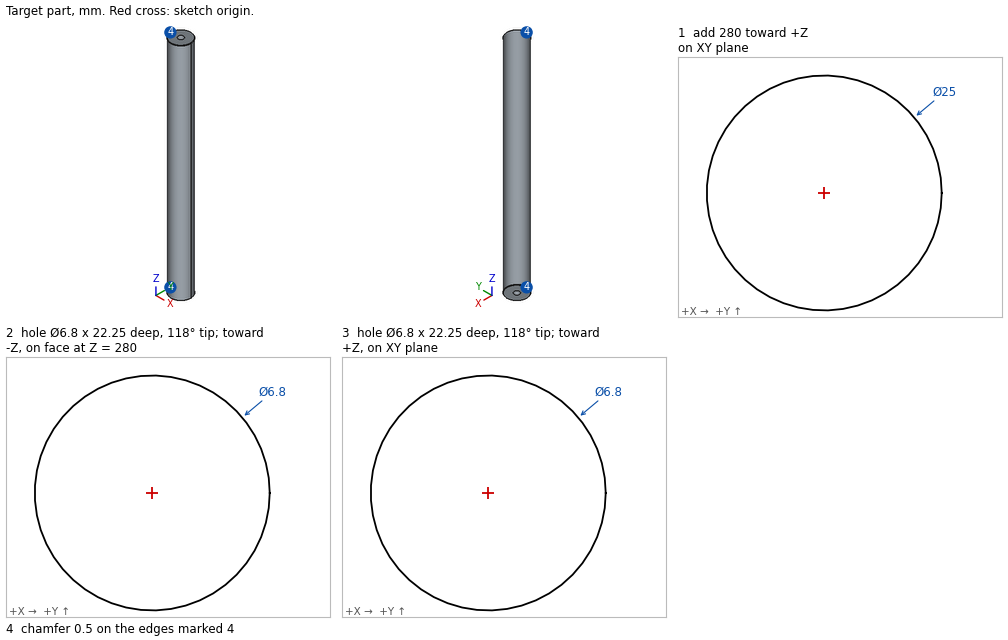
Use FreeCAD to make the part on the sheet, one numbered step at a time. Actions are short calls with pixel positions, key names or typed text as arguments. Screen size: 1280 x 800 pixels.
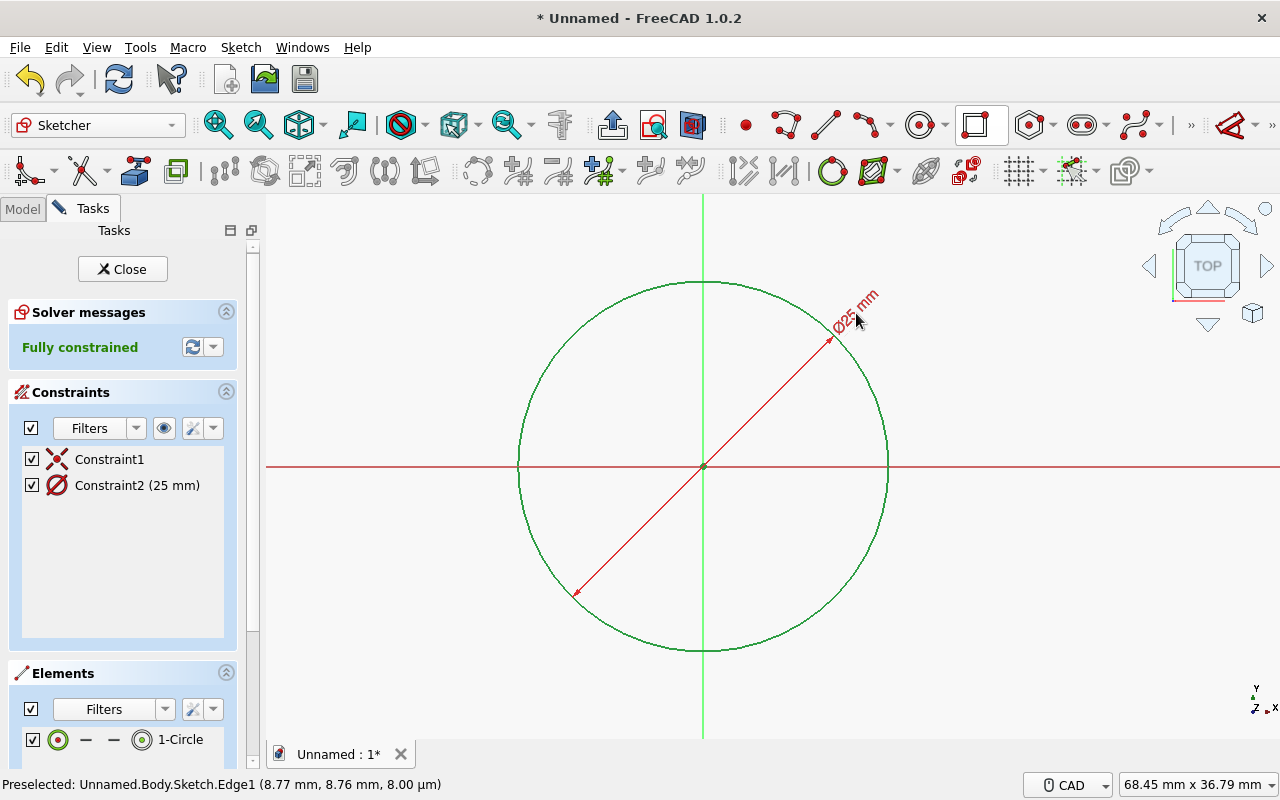
click(123, 269)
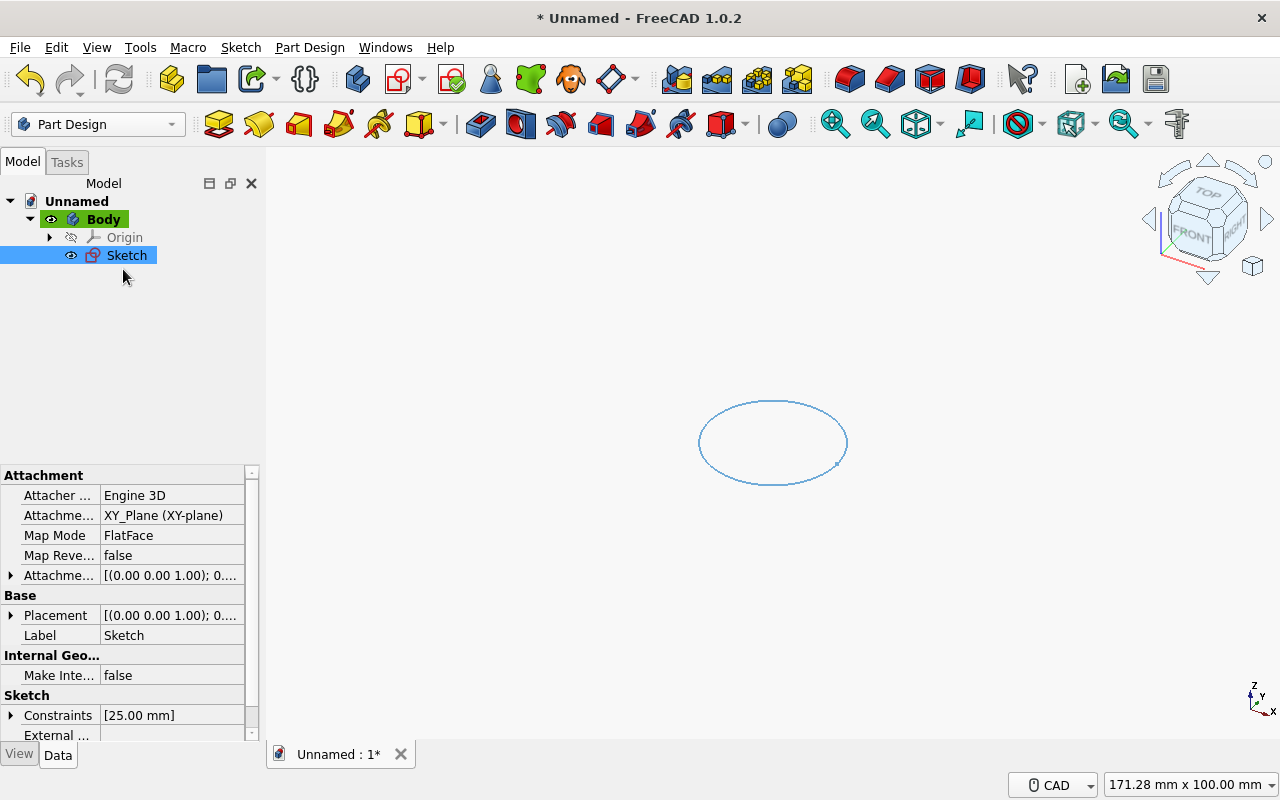
click(220, 124)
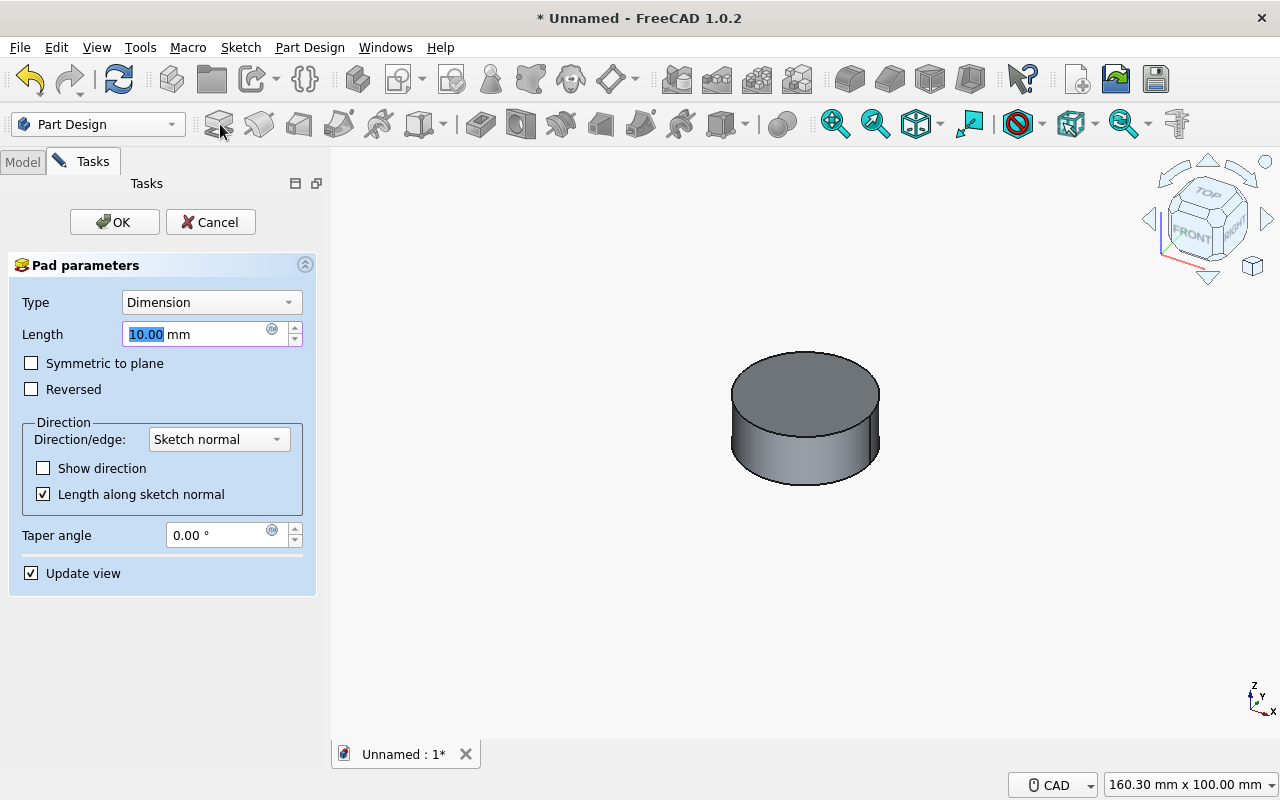
text(280)
key(Tab)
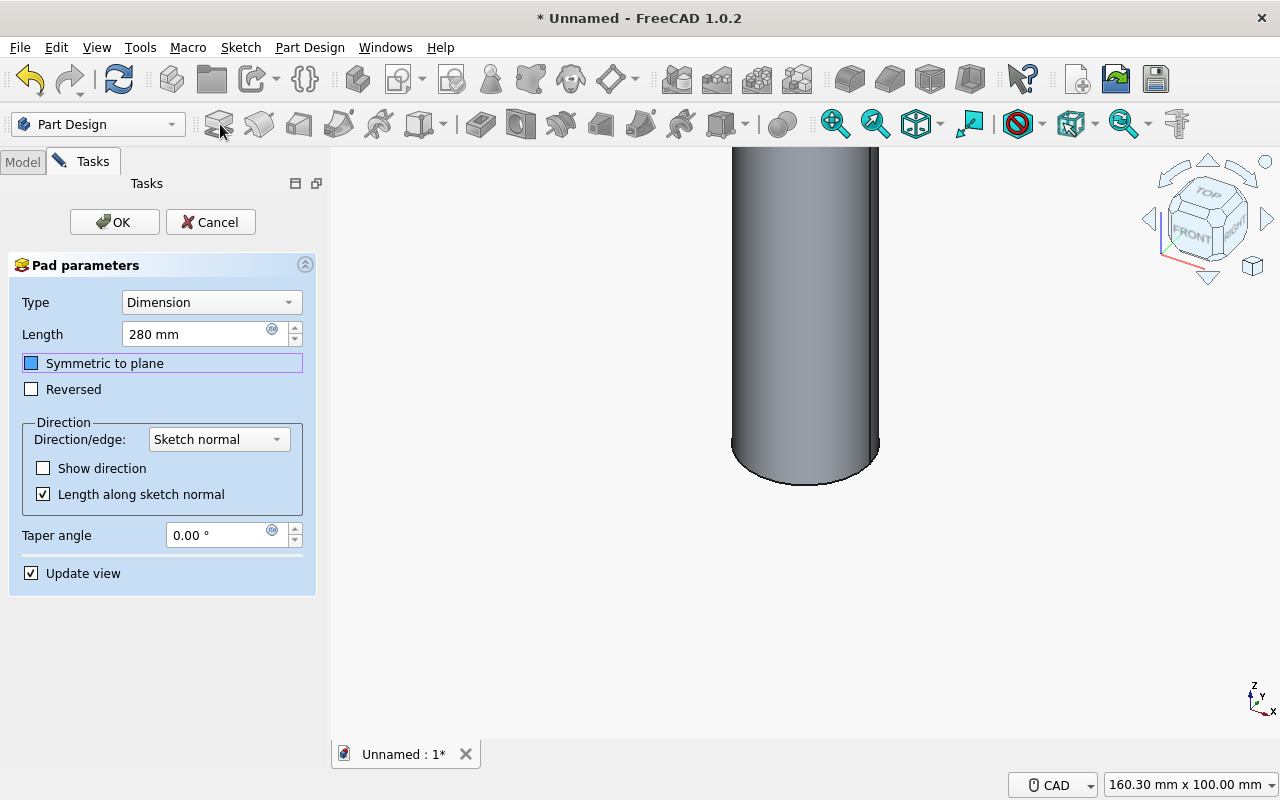
click(115, 222)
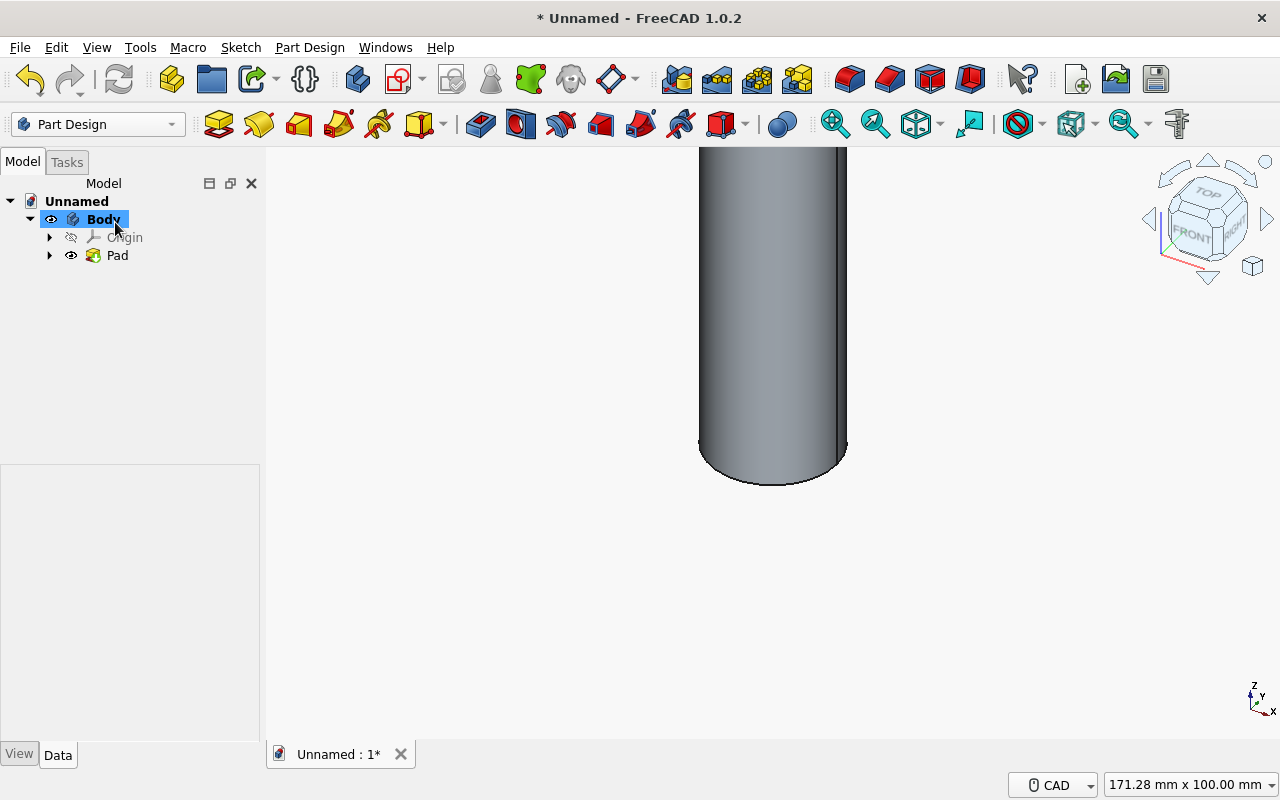
click(836, 124)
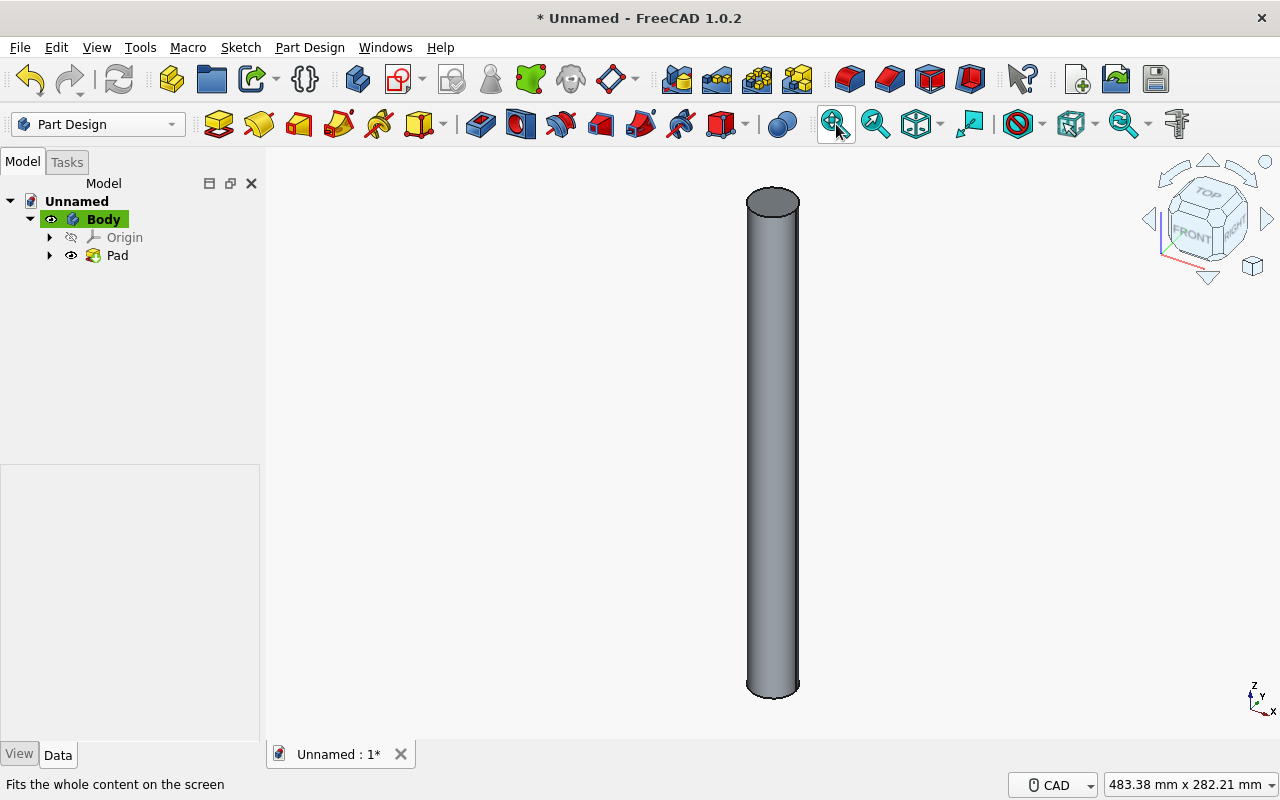
click(773, 201)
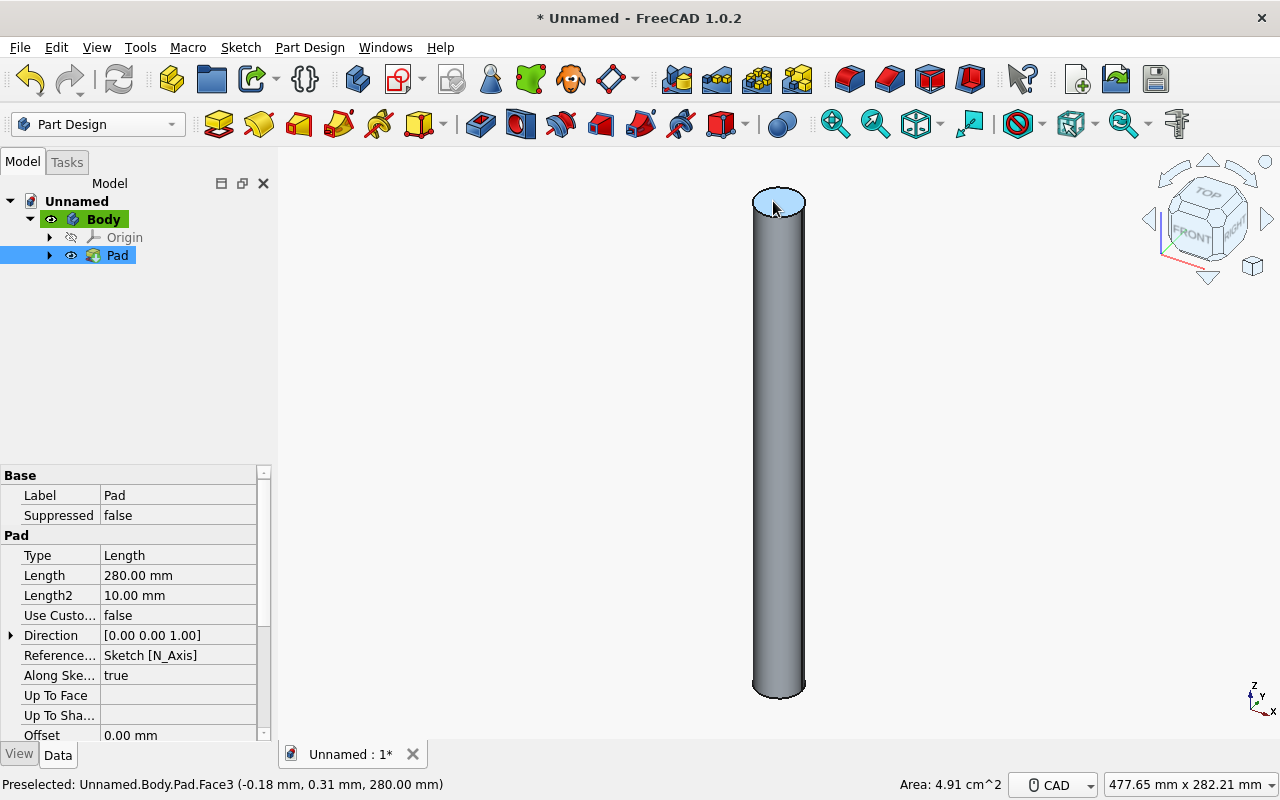
click(398, 80)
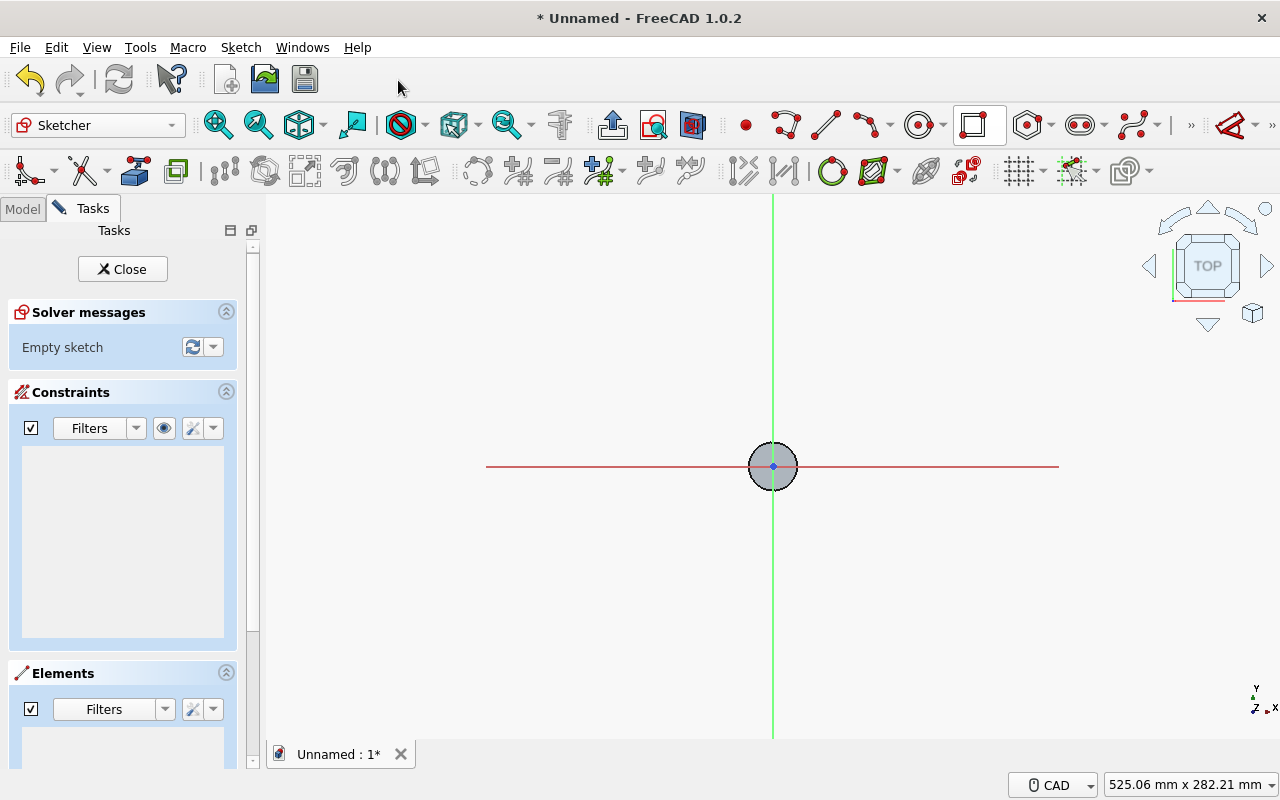
scroll(777, 466, up, 15)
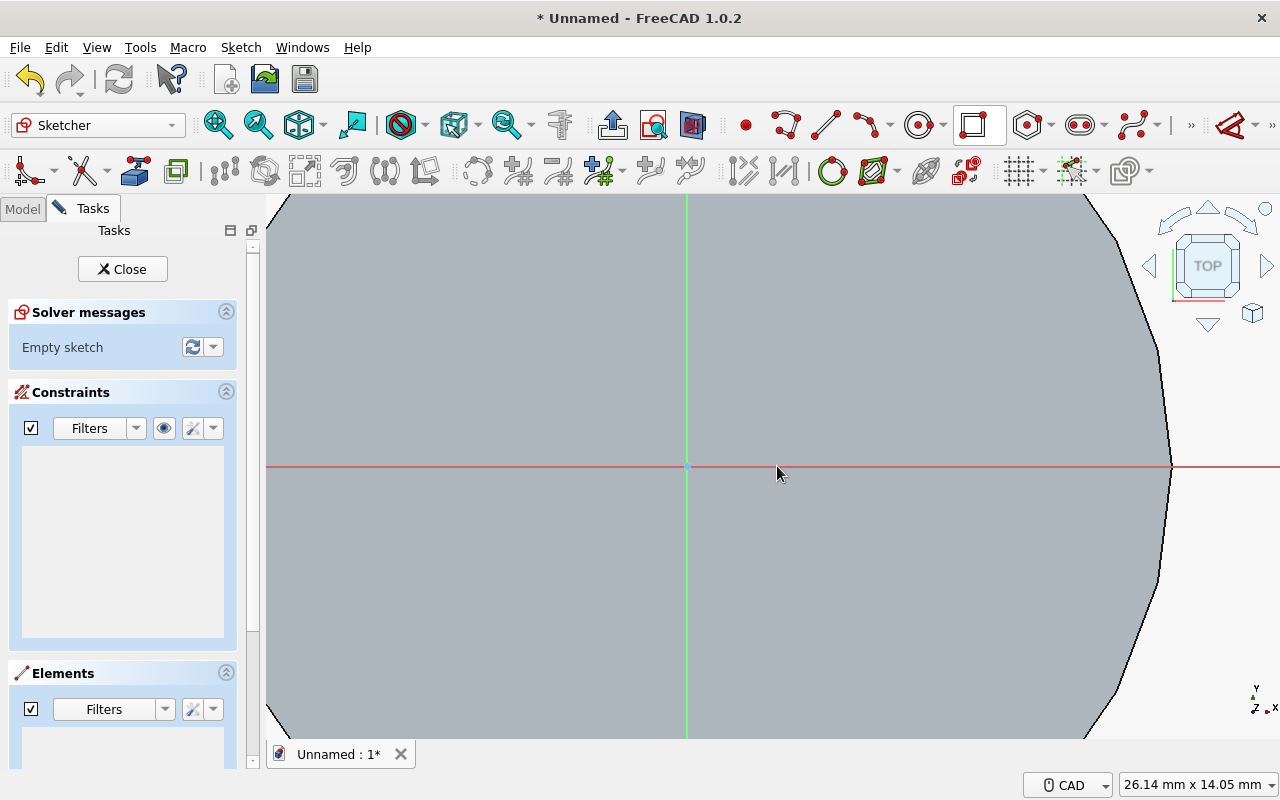
click(920, 126)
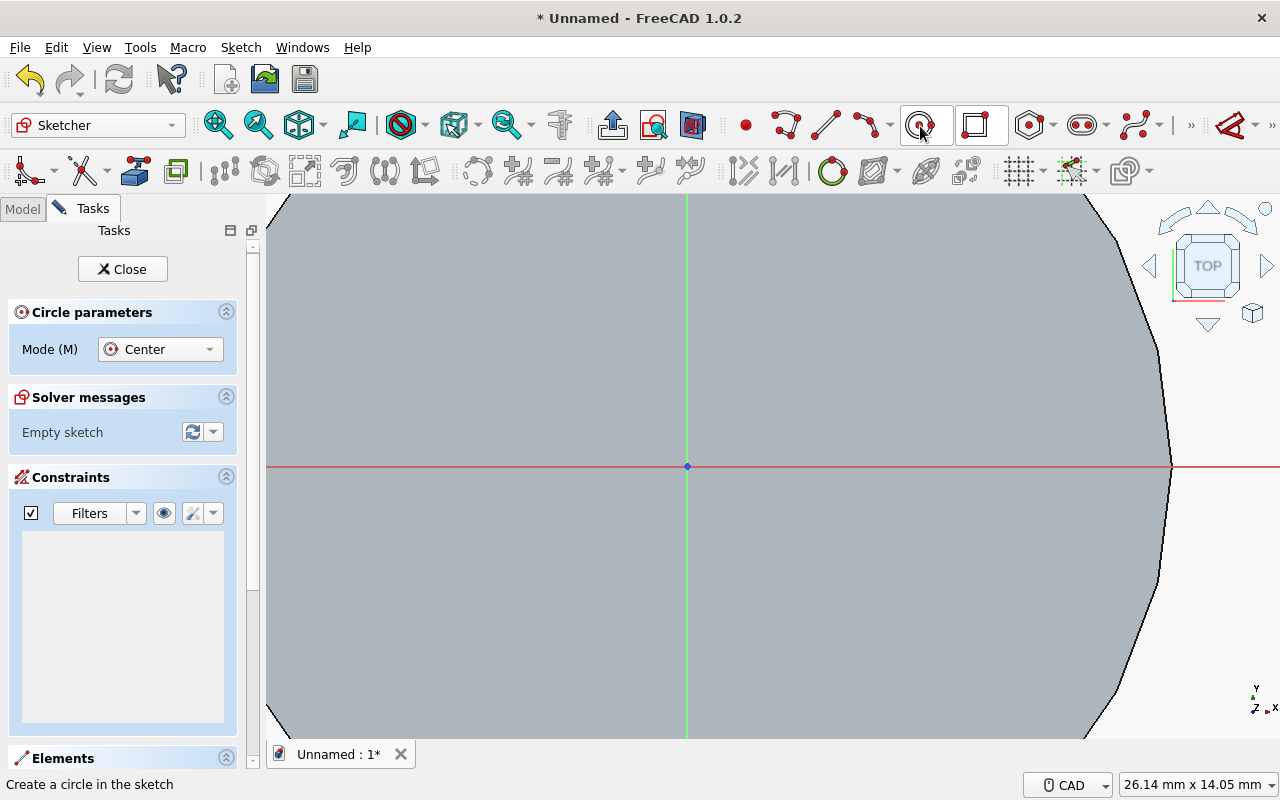
click(687, 466)
click(780, 373)
key(Escape)